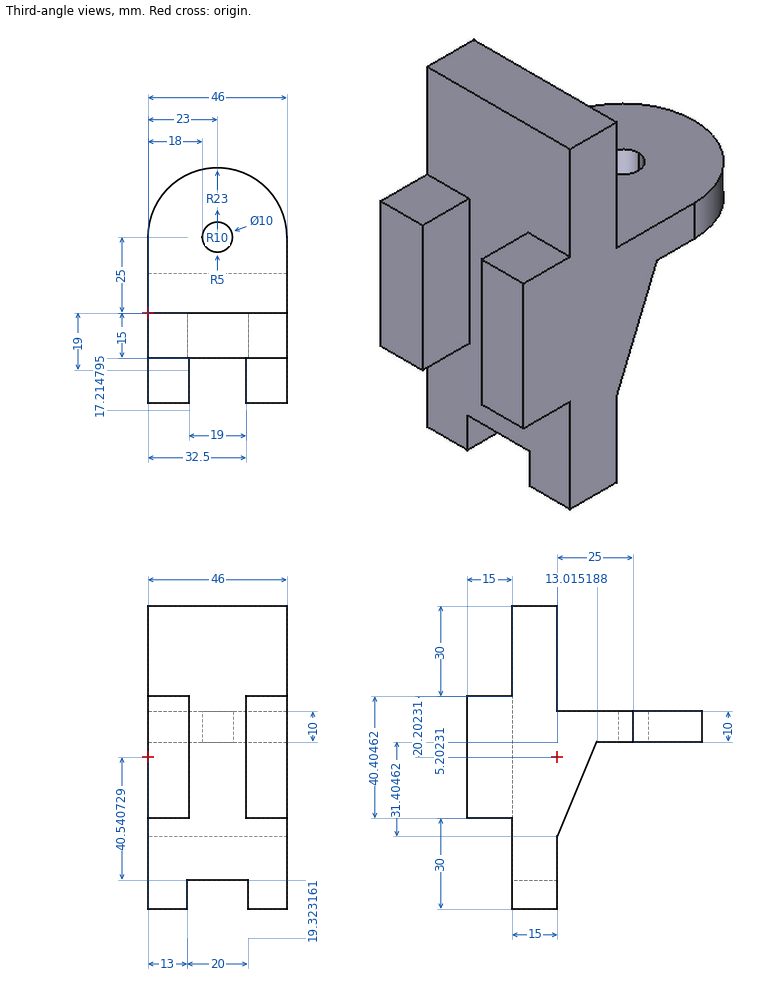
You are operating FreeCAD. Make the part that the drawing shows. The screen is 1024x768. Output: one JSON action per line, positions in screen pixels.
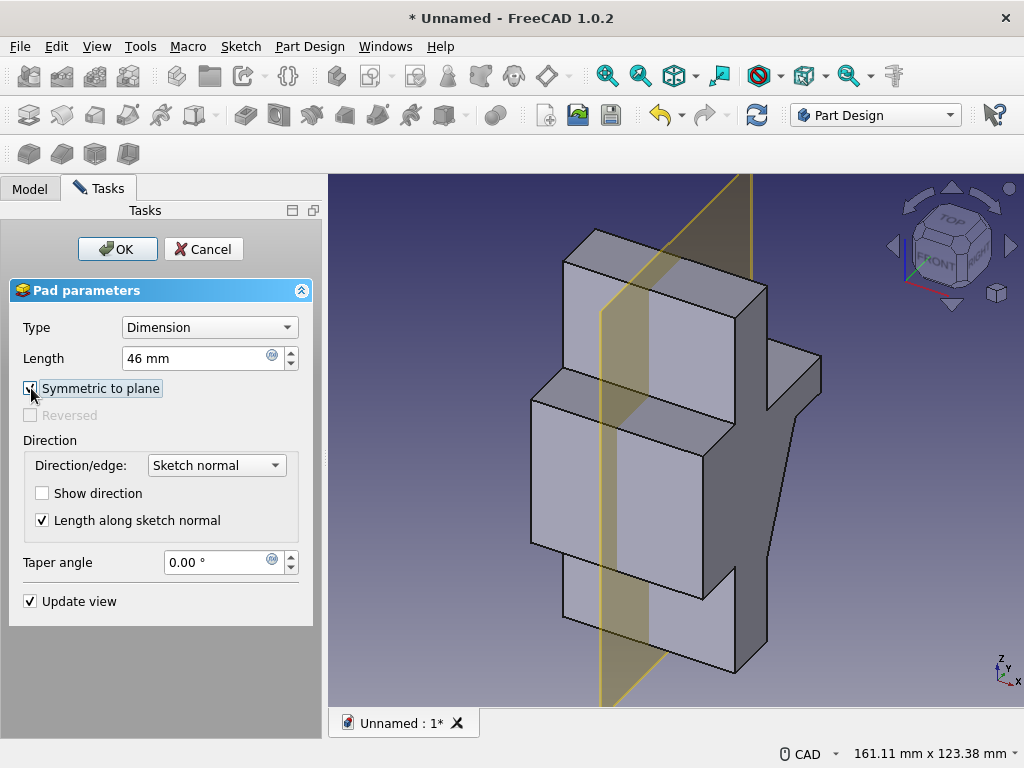
{"action": "left_click", "coordinate": [118, 249]}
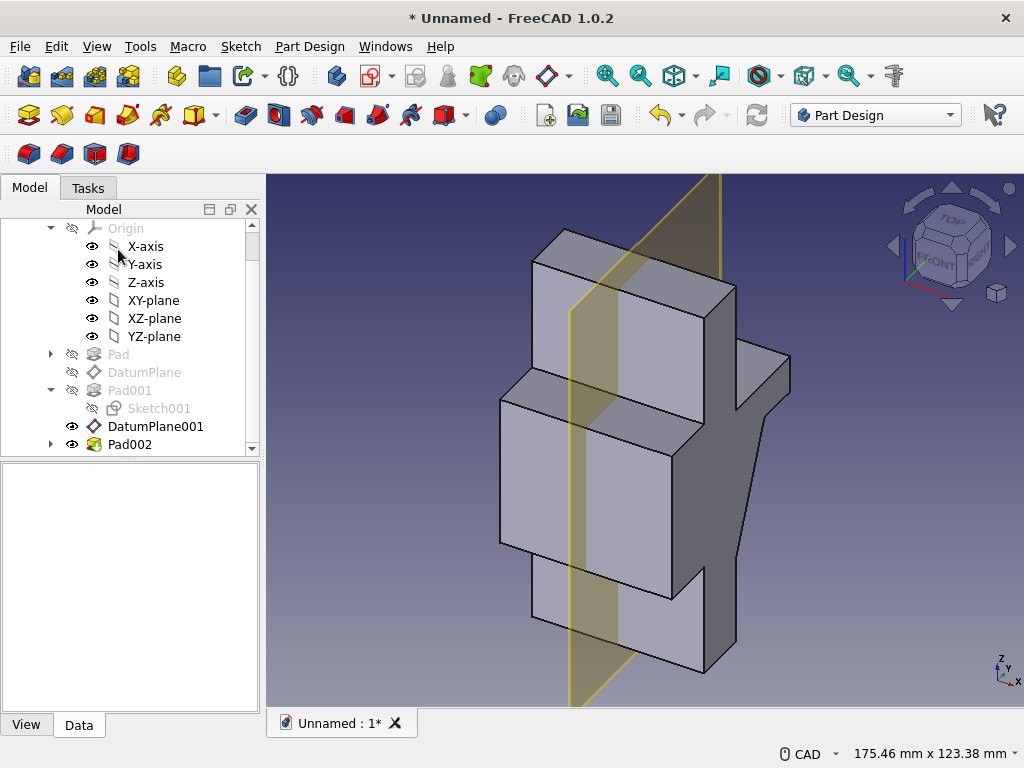
{"action": "left_click", "coordinate": [117, 426]}
{"action": "key", "text": "space"}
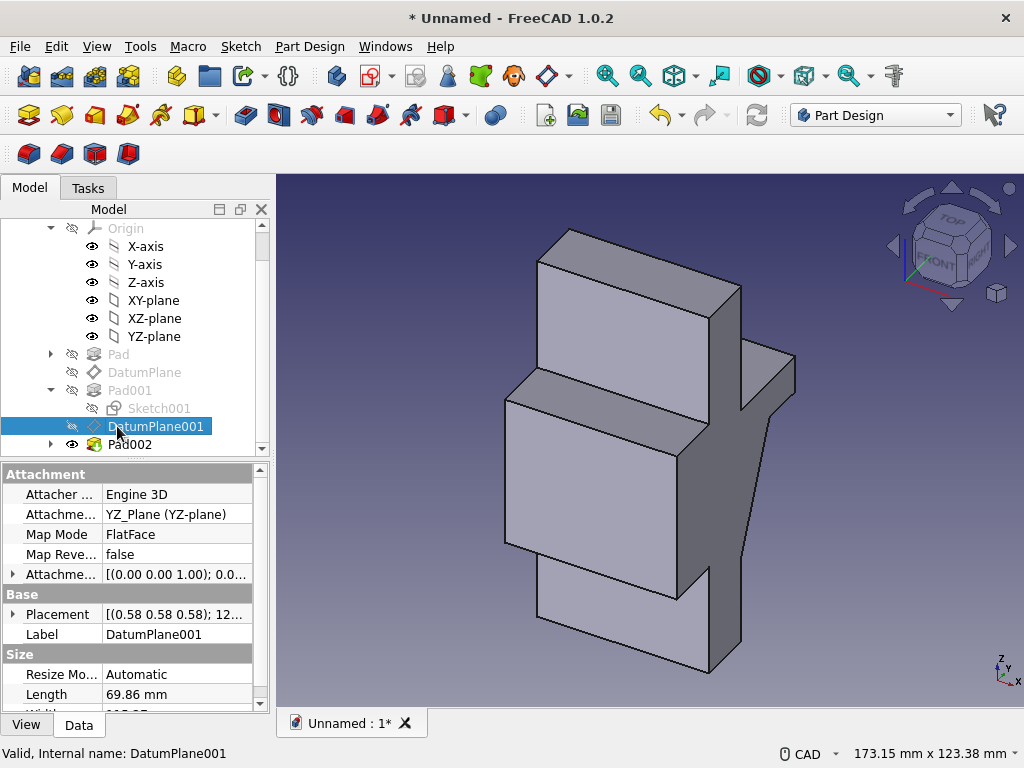
{"action": "key", "text": "5"}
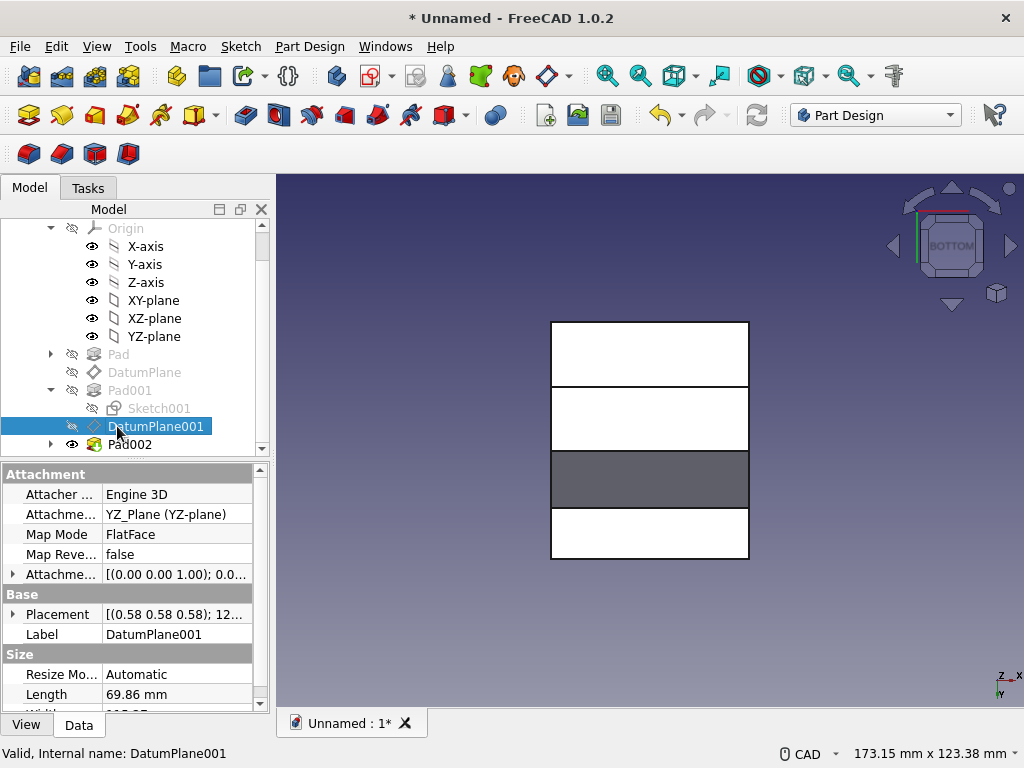
{"action": "left_click", "coordinate": [608, 76]}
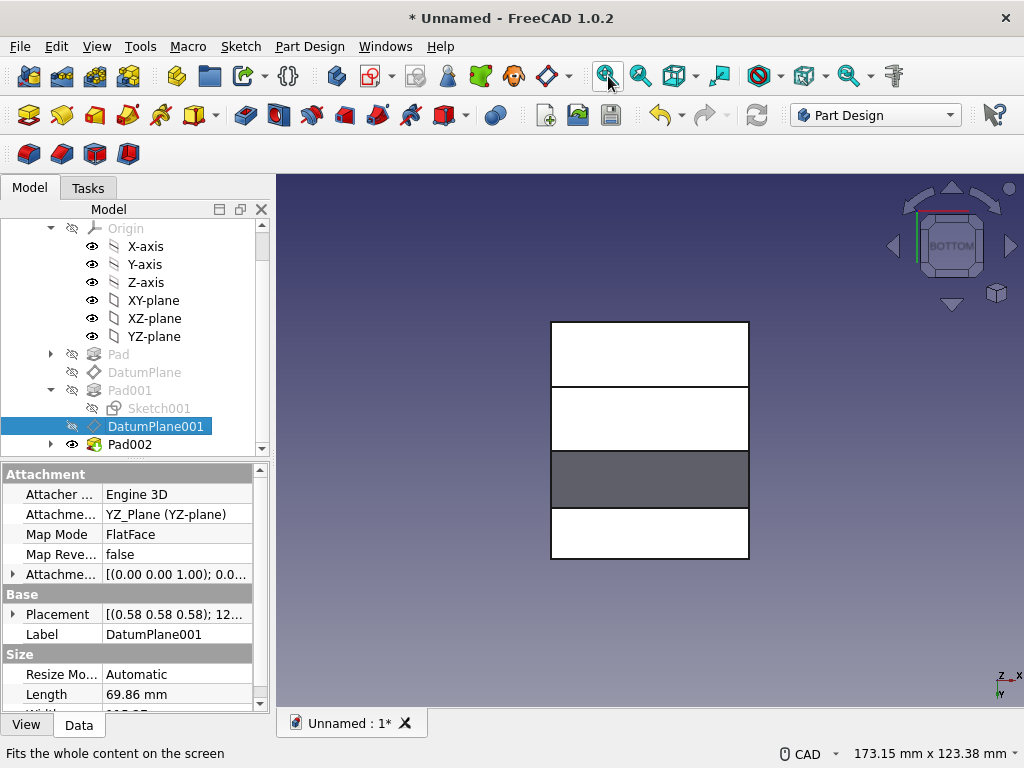
{"action": "left_click", "coordinate": [650, 532]}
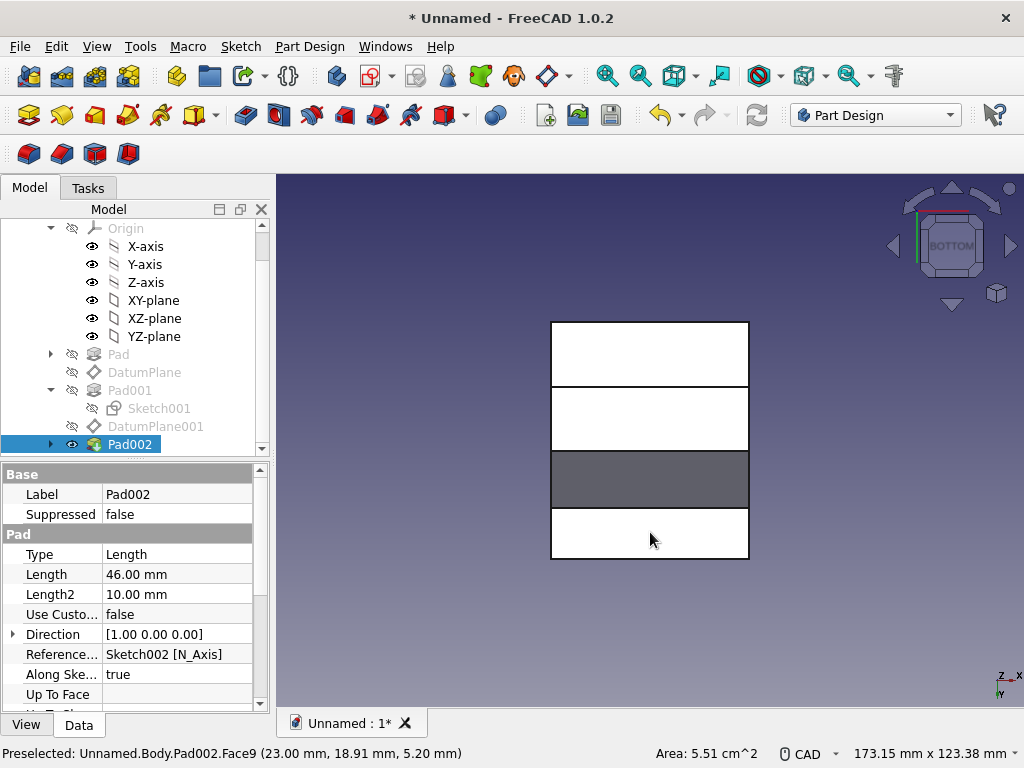
{"action": "left_click", "coordinate": [370, 76]}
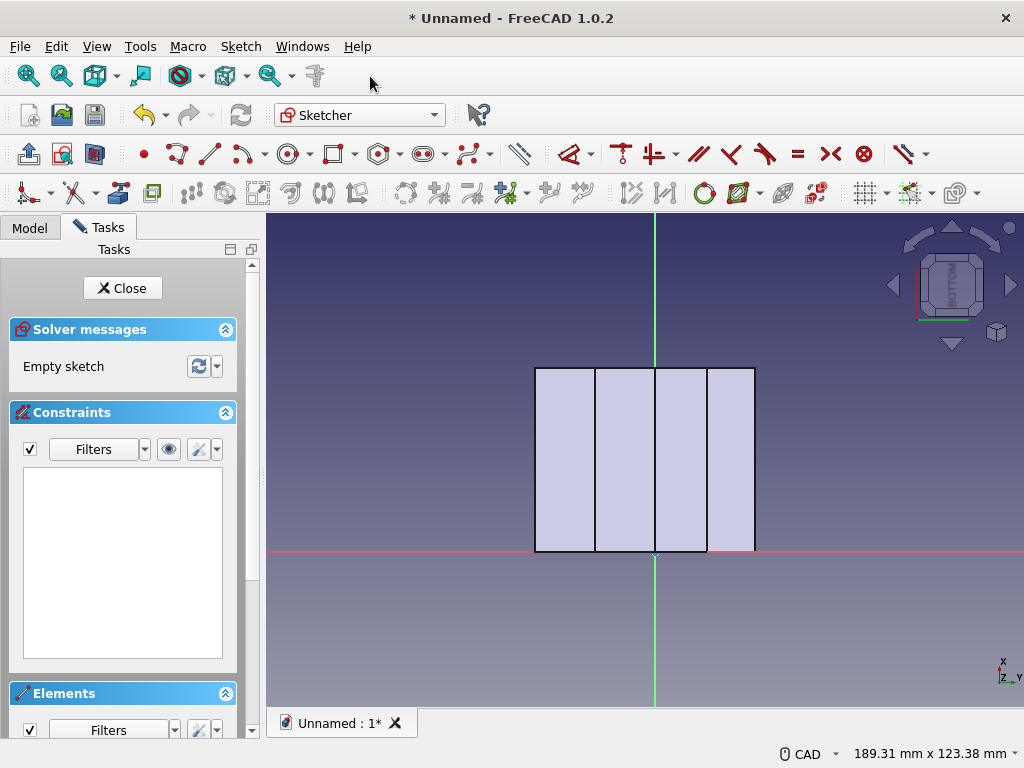
{"action": "scroll", "coordinate": [576, 460], "scroll_direction": "down", "scroll_amount": 5}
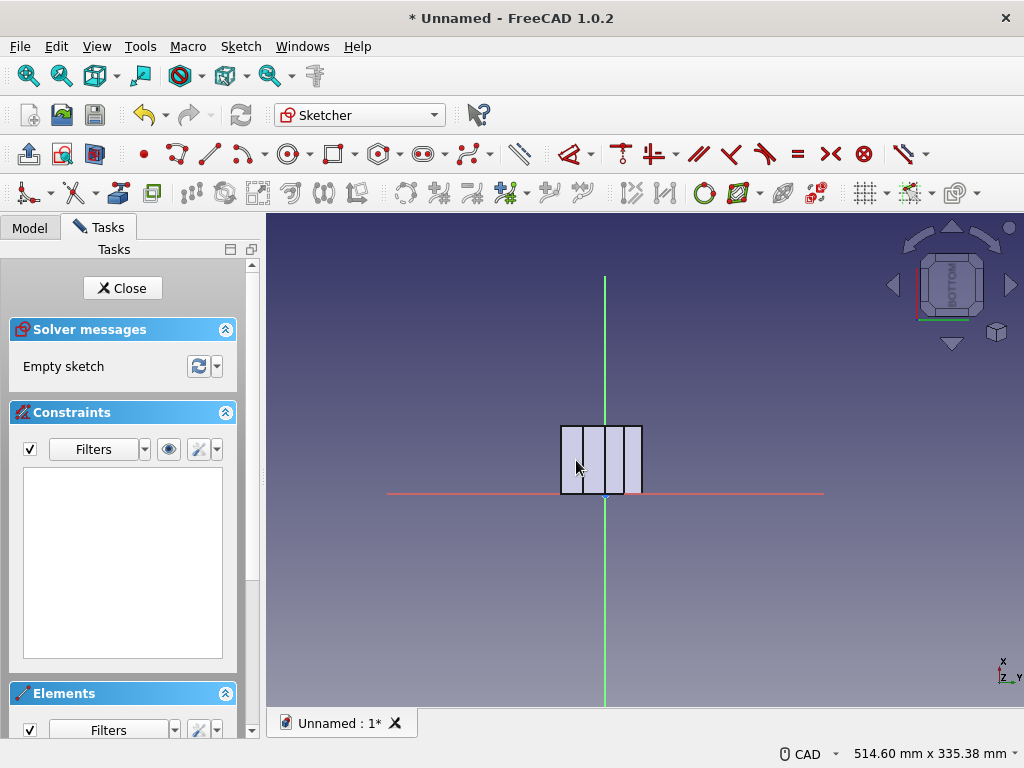
{"action": "scroll", "coordinate": [657, 460], "scroll_direction": "up", "scroll_amount": 8}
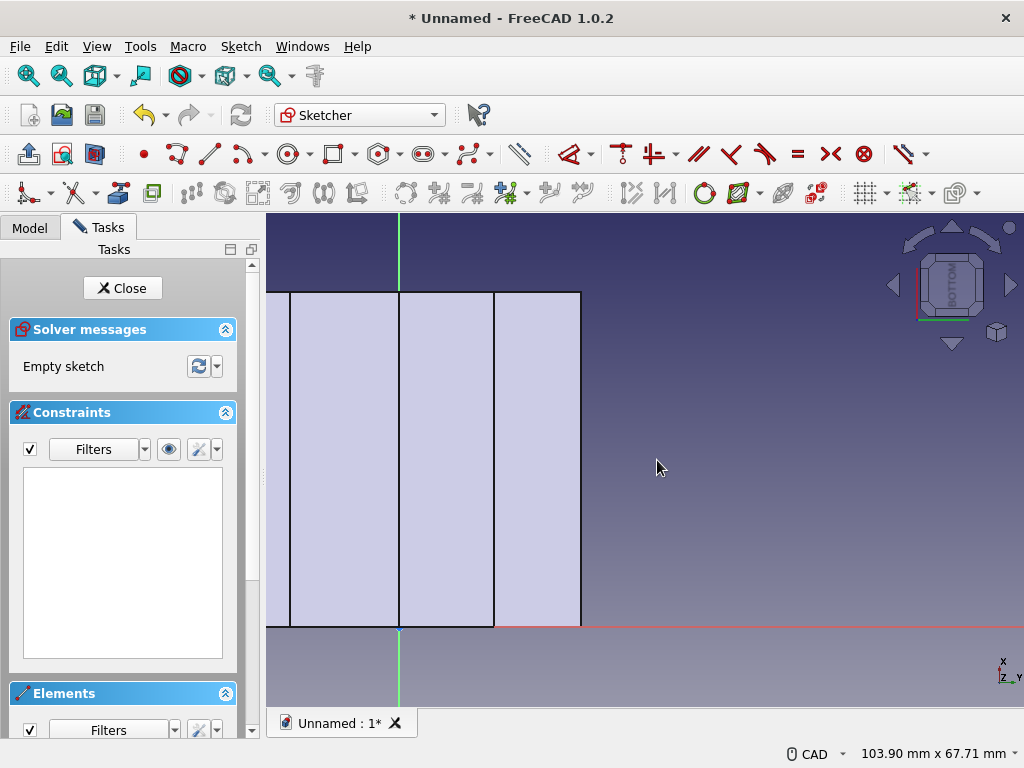
{"action": "key", "text": "g l"}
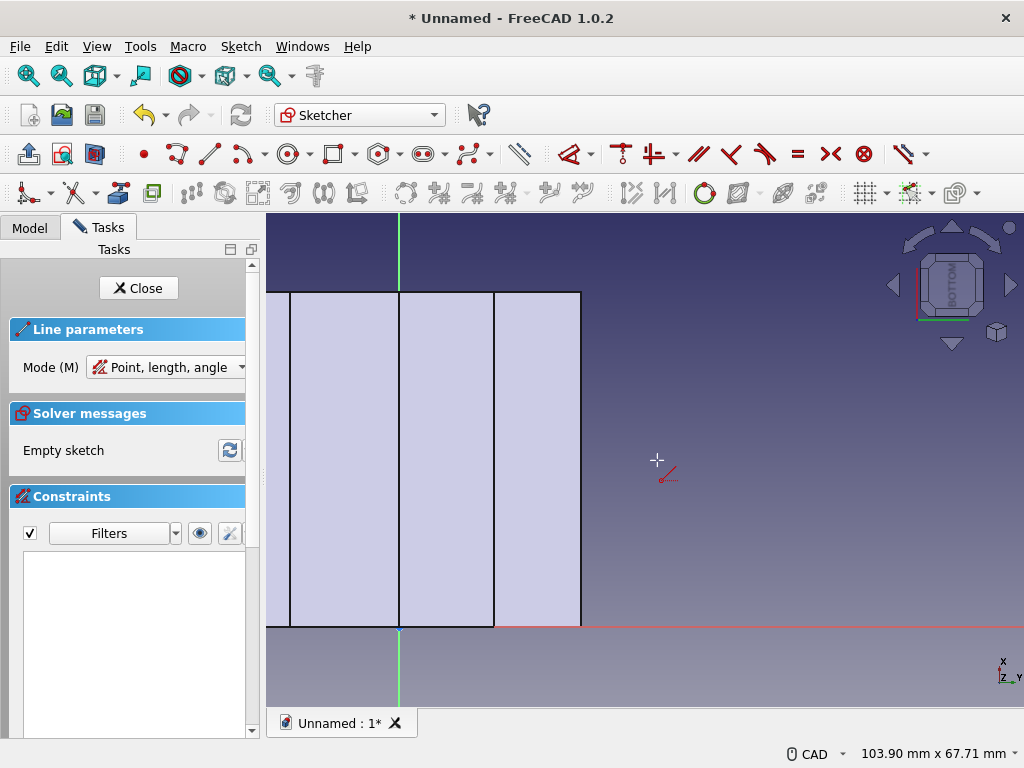
{"action": "left_click", "coordinate": [581, 533]}
{"action": "left_click", "coordinate": [581, 627]}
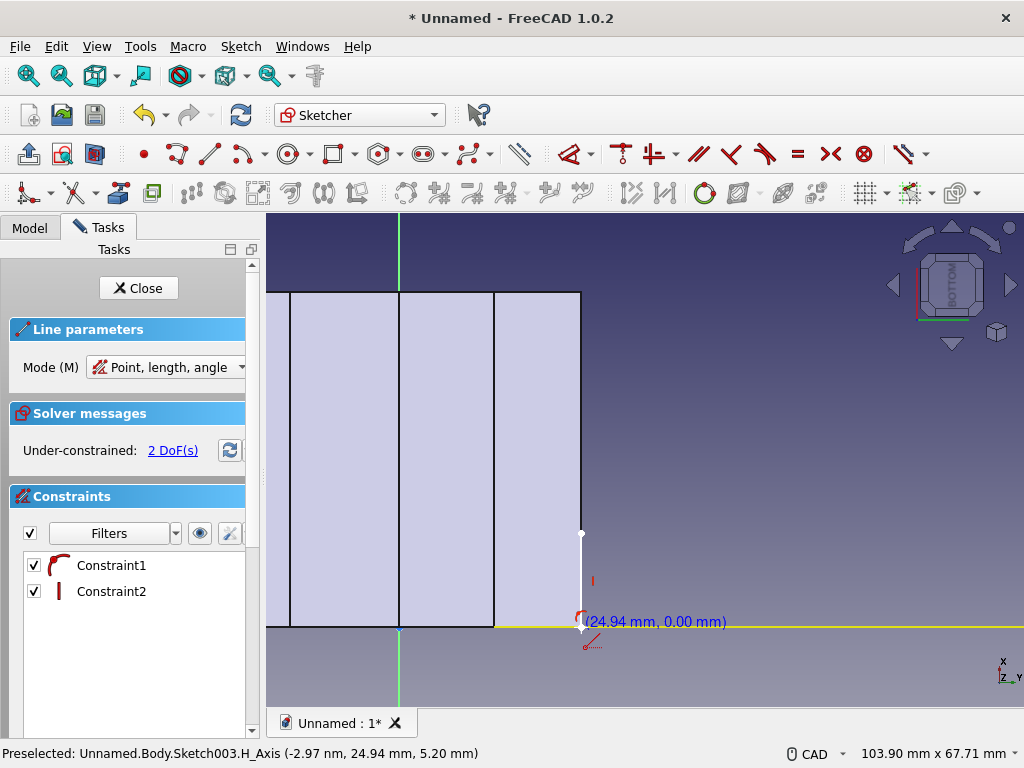
{"action": "left_click", "coordinate": [581, 292]}
{"action": "left_click", "coordinate": [581, 387]}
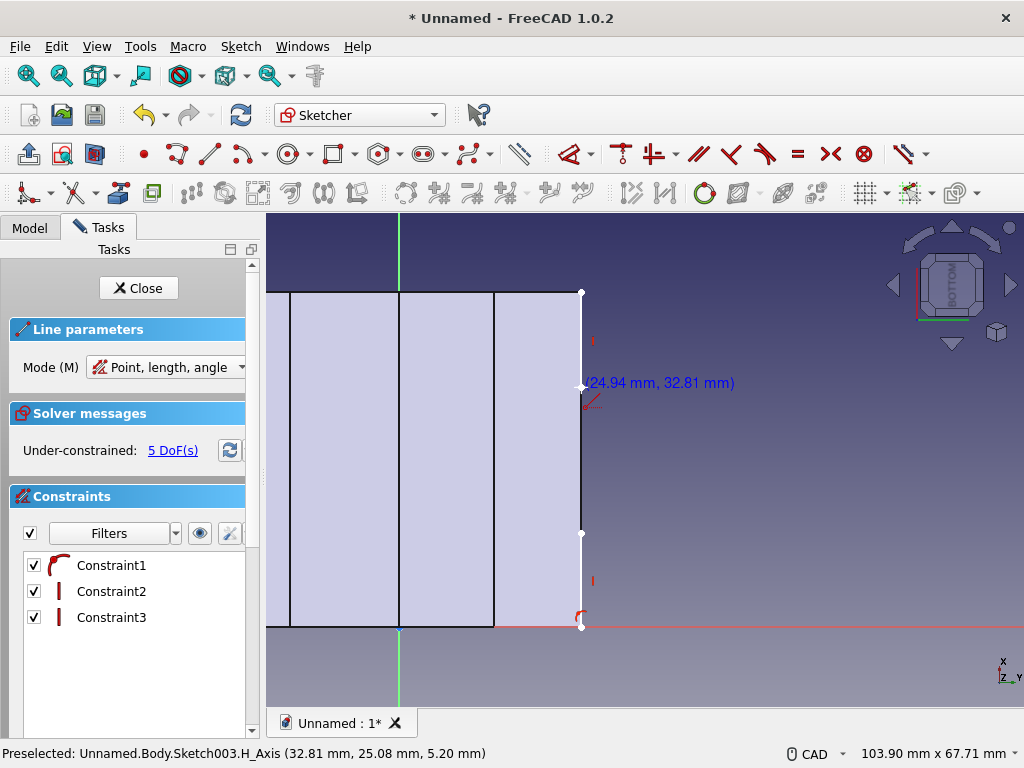
{"action": "key", "text": "g 3 a"}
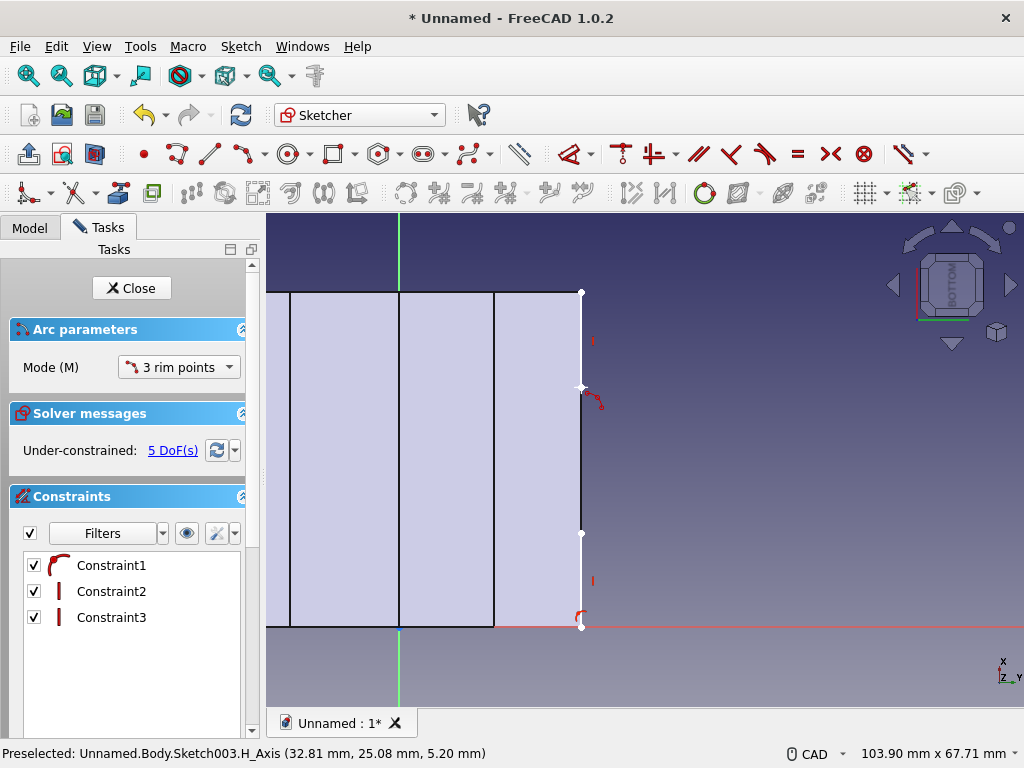
{"action": "left_click", "coordinate": [581, 627]}
{"action": "left_click", "coordinate": [581, 293]}
{"action": "left_click", "coordinate": [749, 460]}